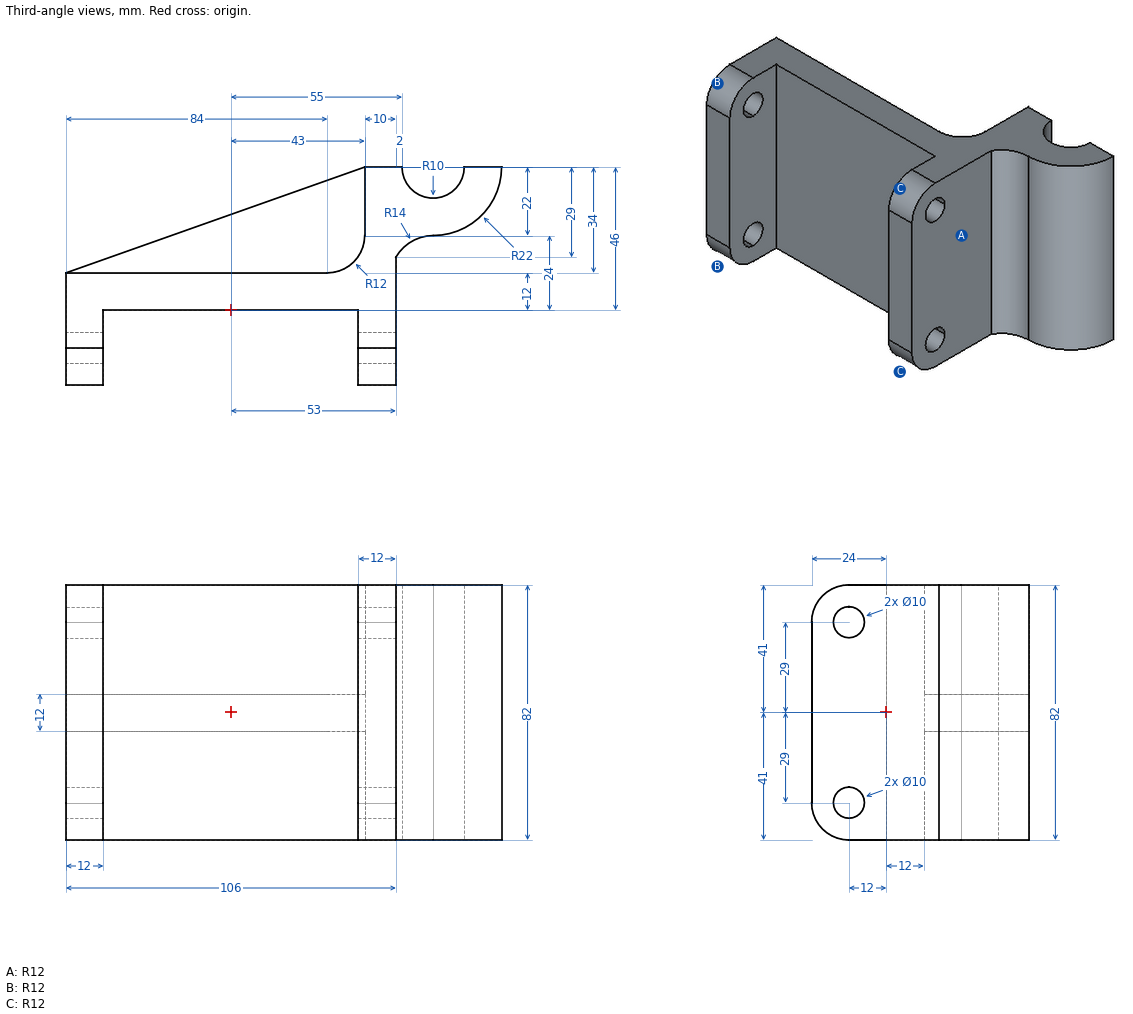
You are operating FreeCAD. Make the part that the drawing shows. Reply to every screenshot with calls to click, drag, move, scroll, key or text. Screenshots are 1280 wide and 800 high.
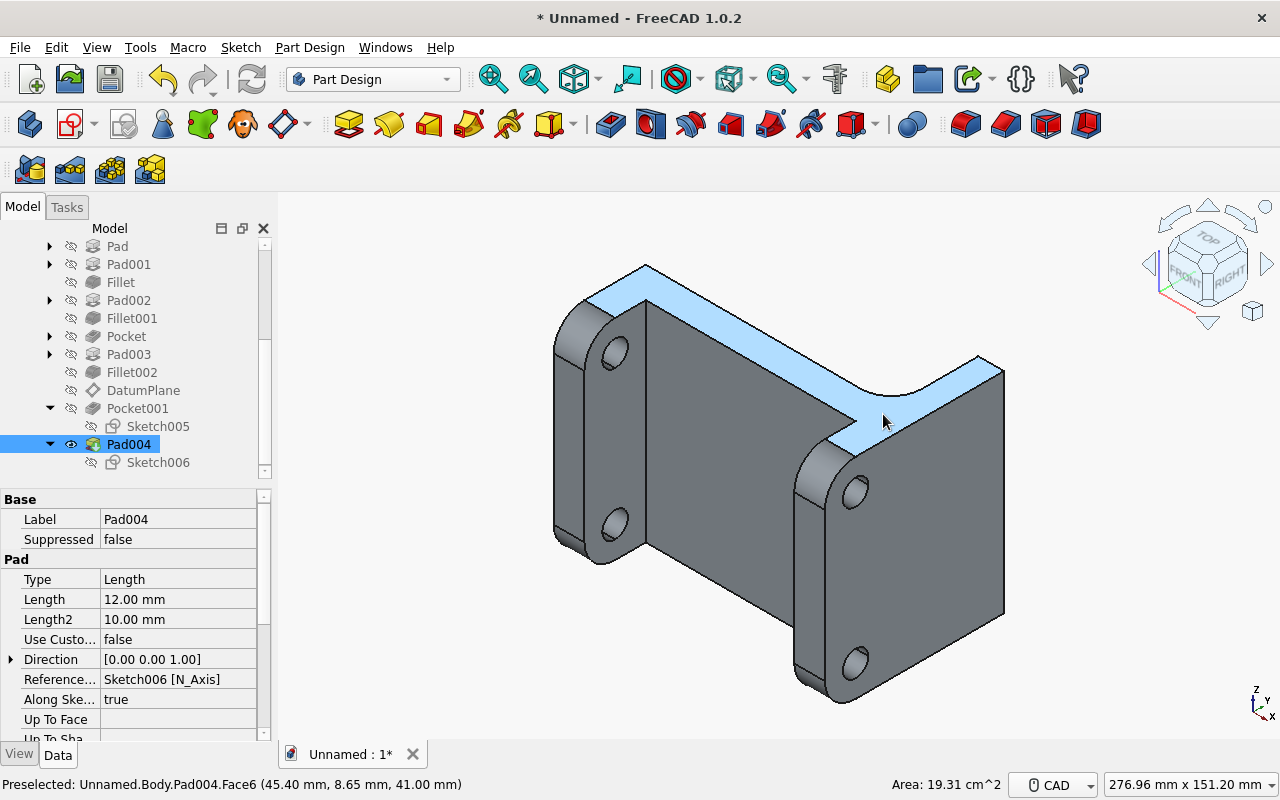
click(70, 124)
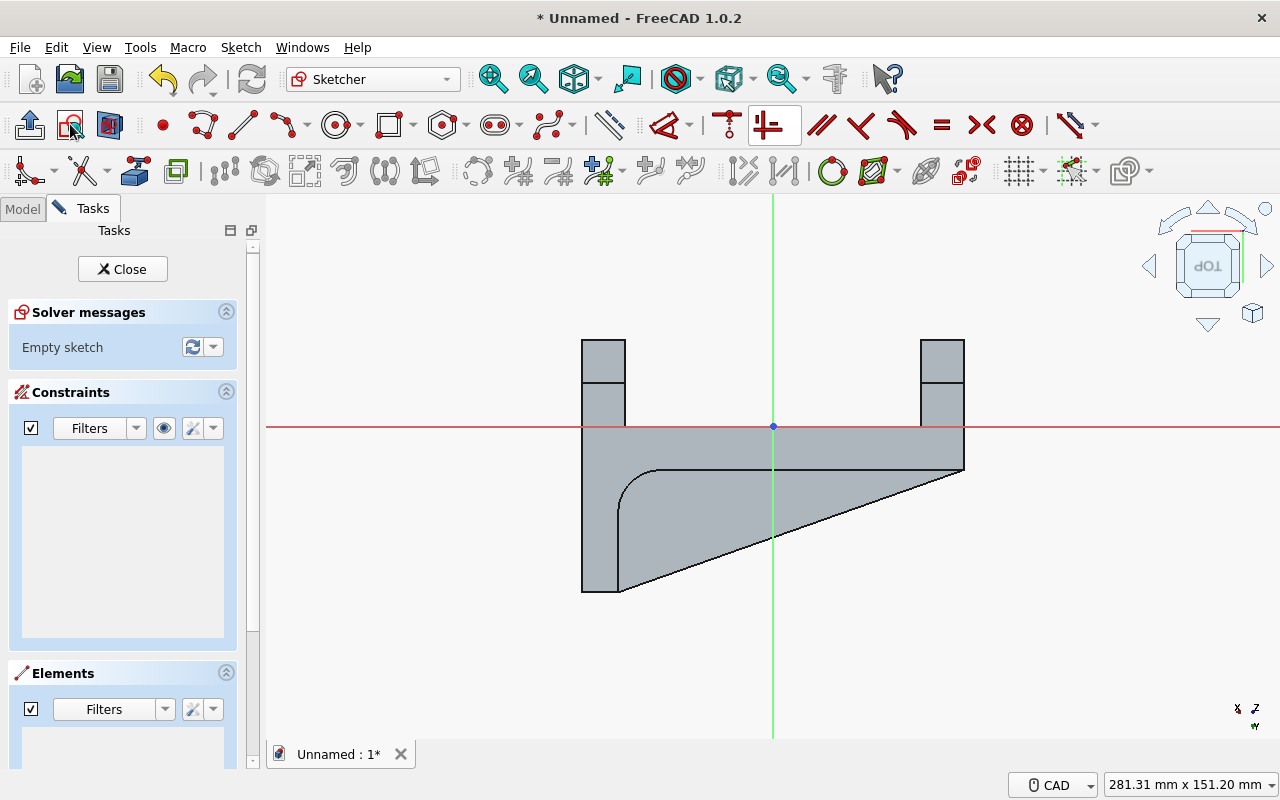
scroll(441, 572, up, 6)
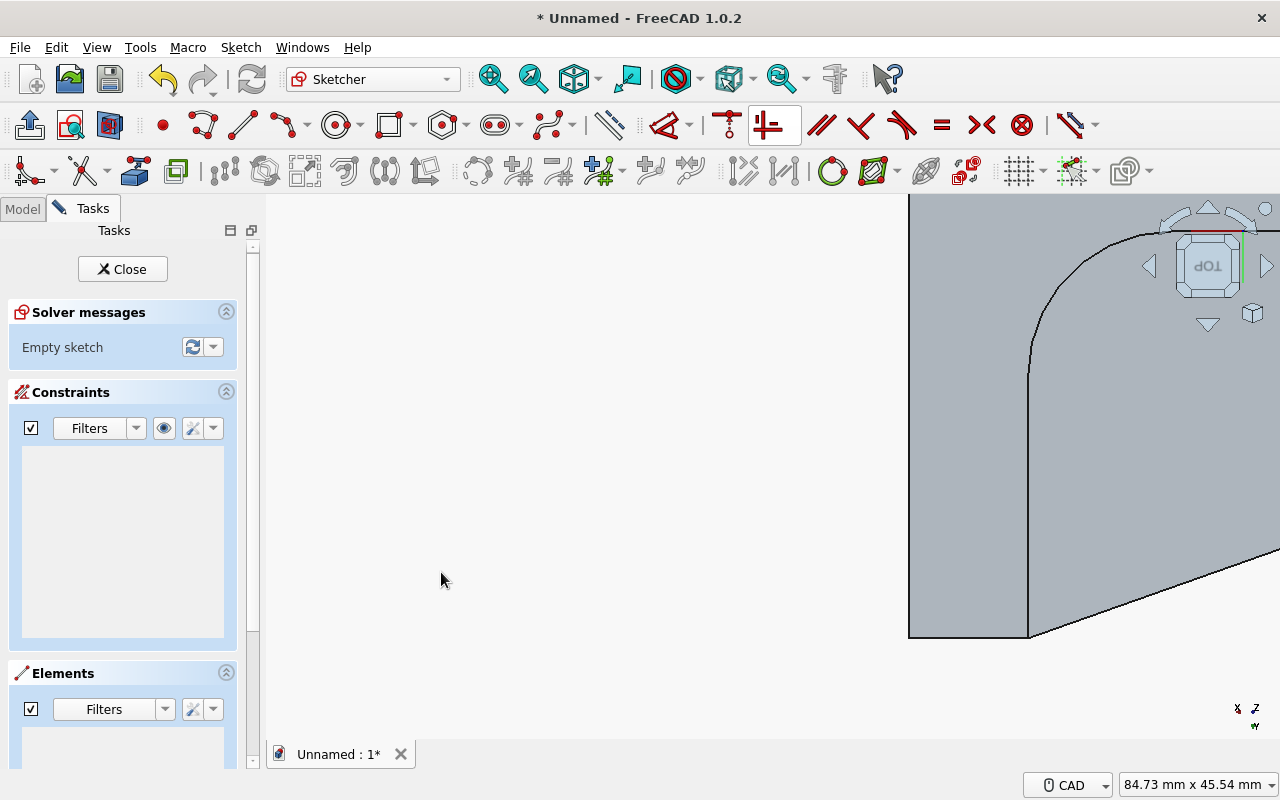
key(g)
key(m)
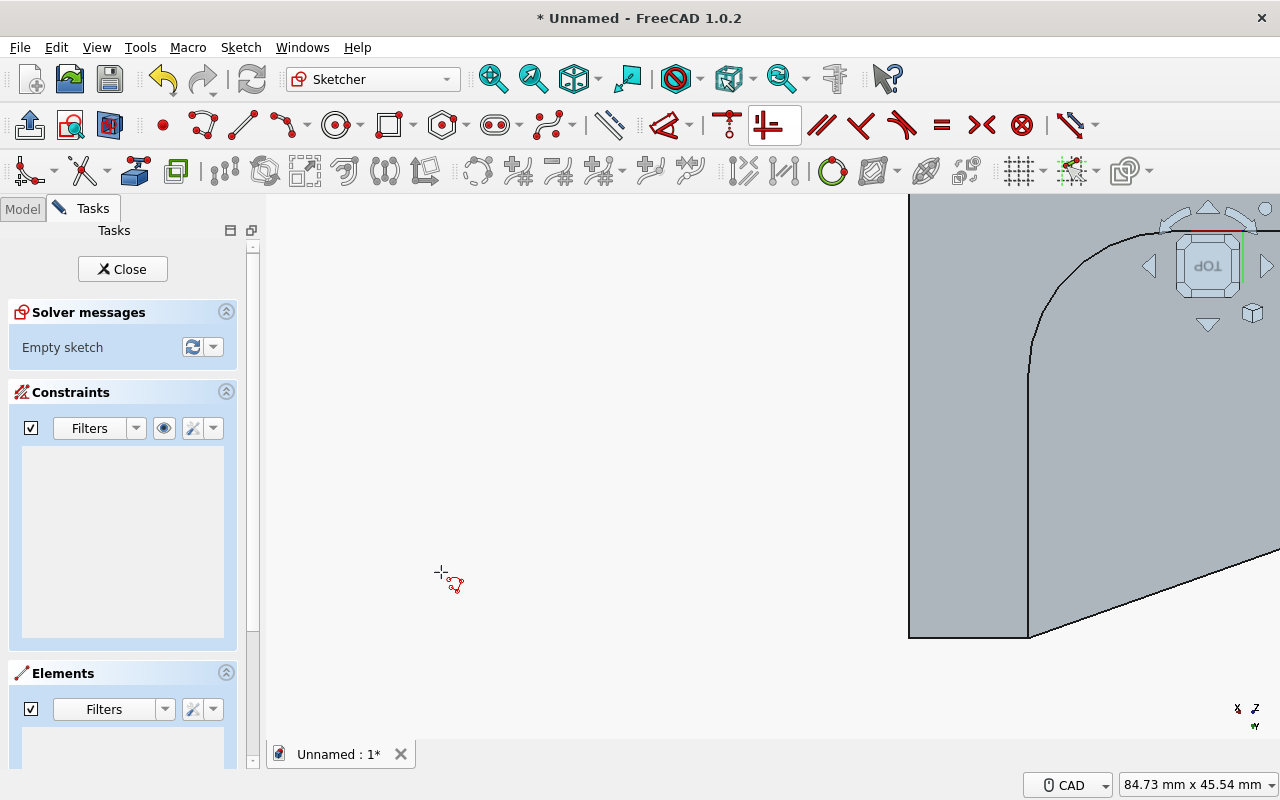
click(885, 638)
click(909, 638)
click(909, 291)
right_click(909, 291)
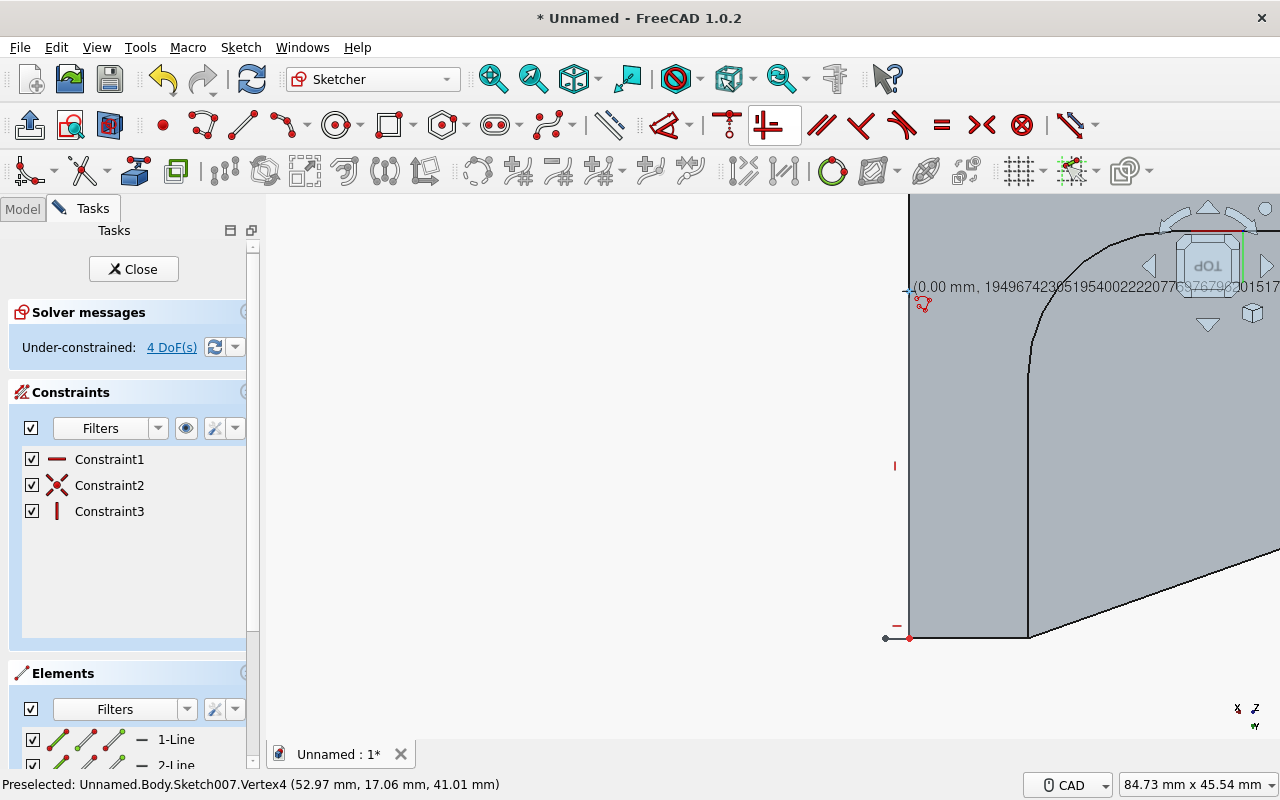
click(244, 126)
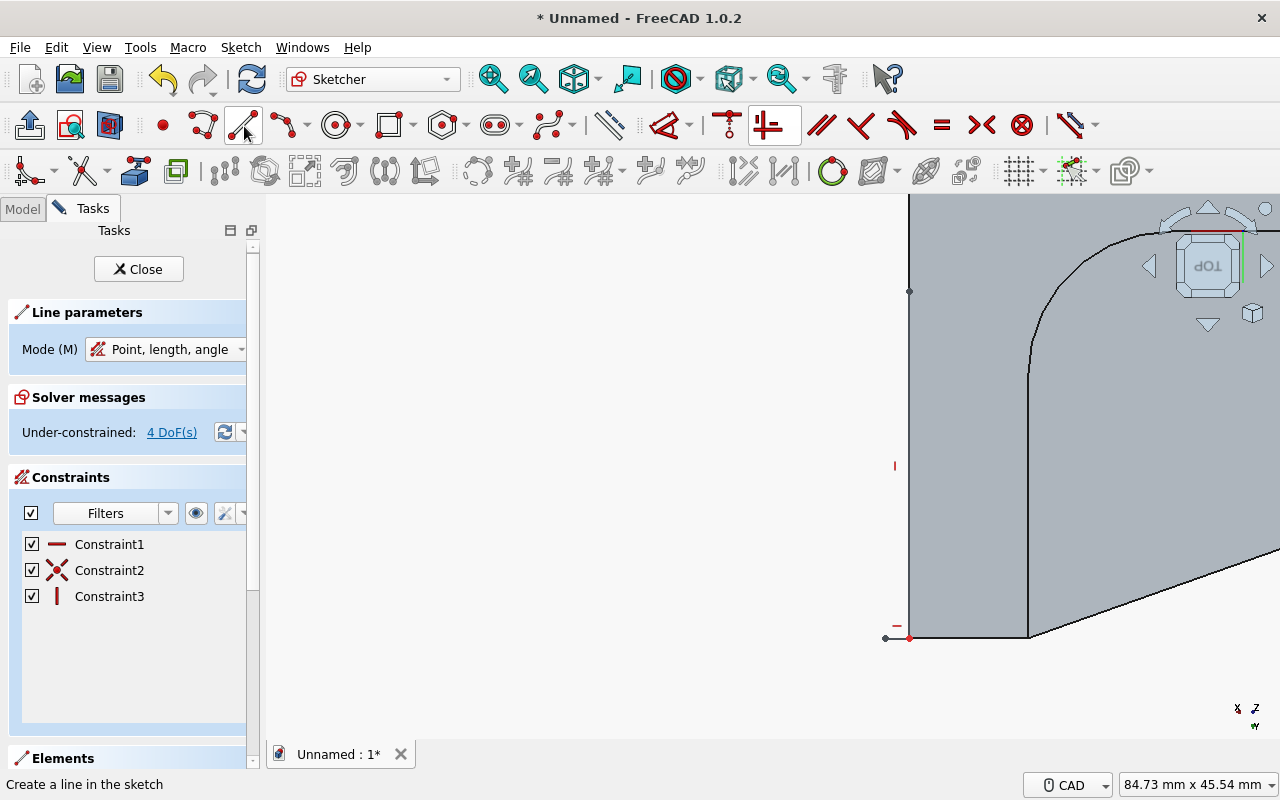
click(502, 638)
click(645, 638)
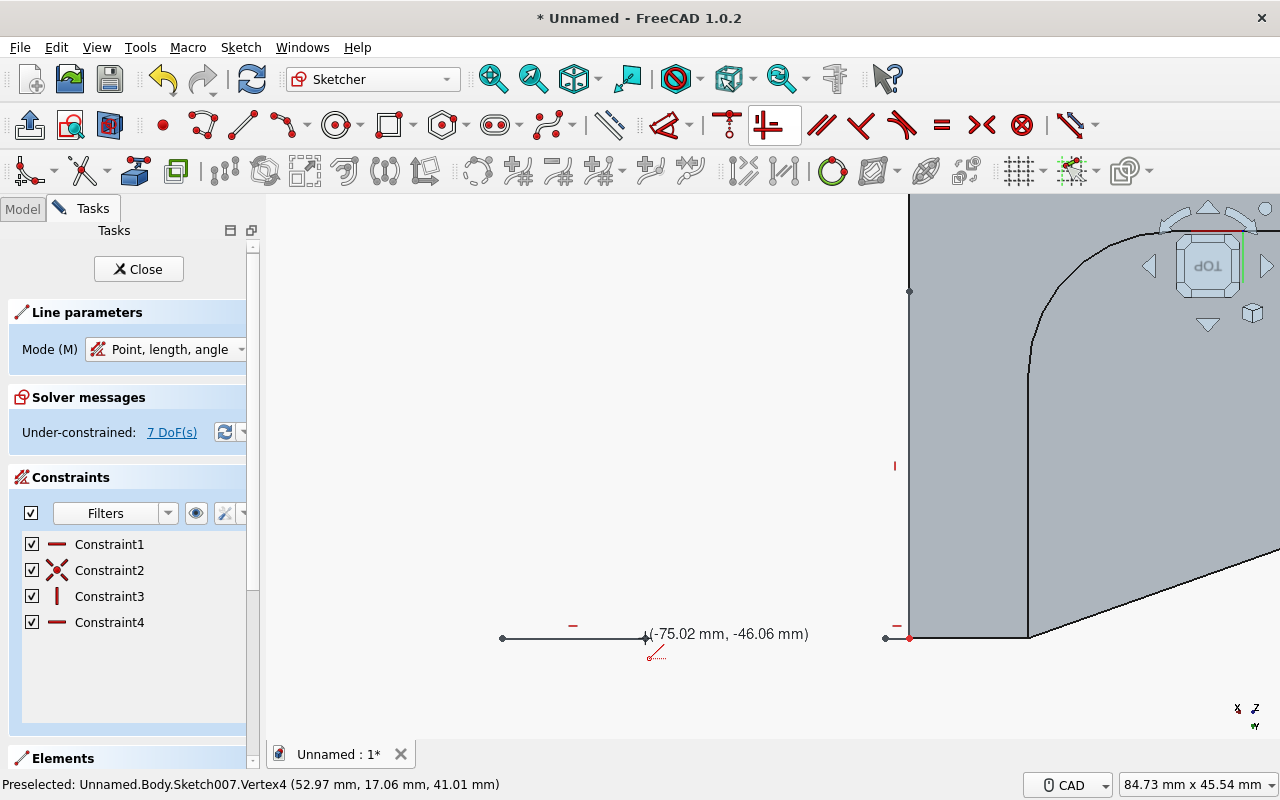
click(284, 126)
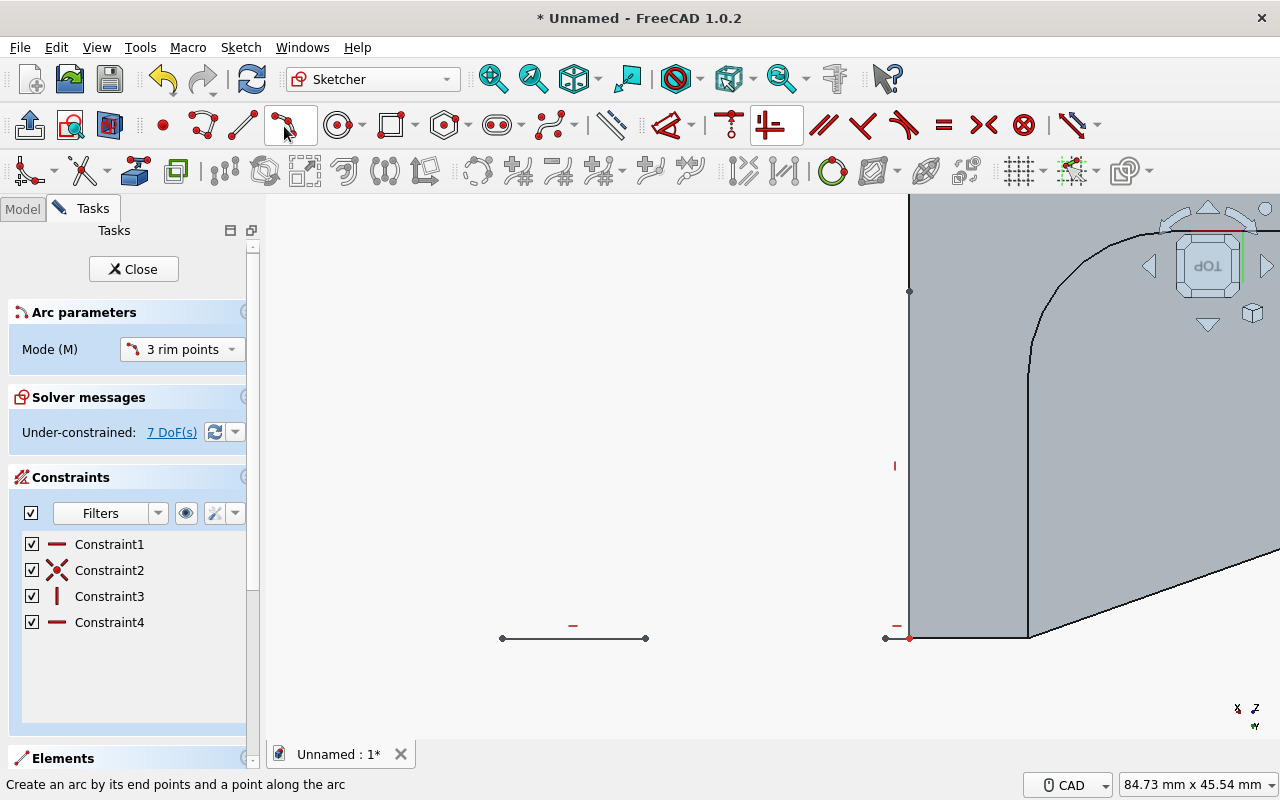
click(909, 292)
click(764, 375)
click(848, 352)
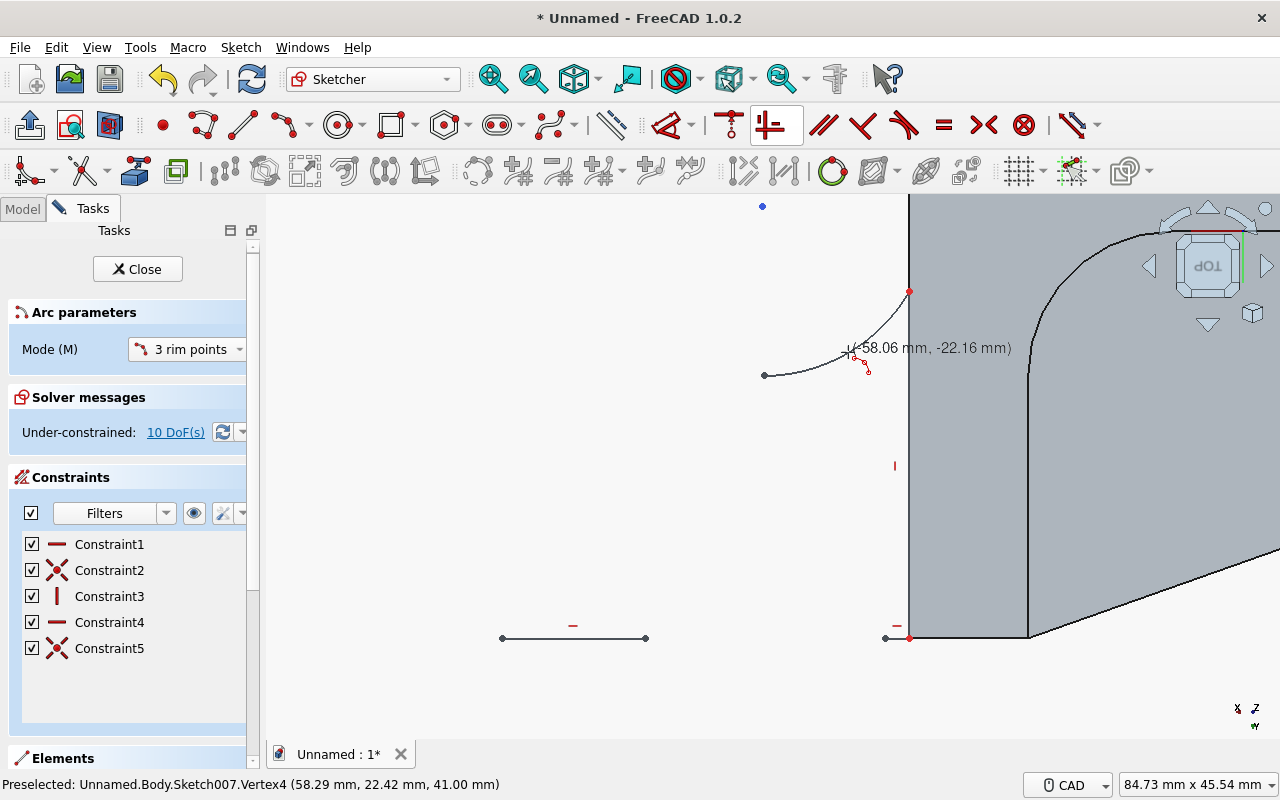
click(764, 376)
click(502, 639)
click(578, 452)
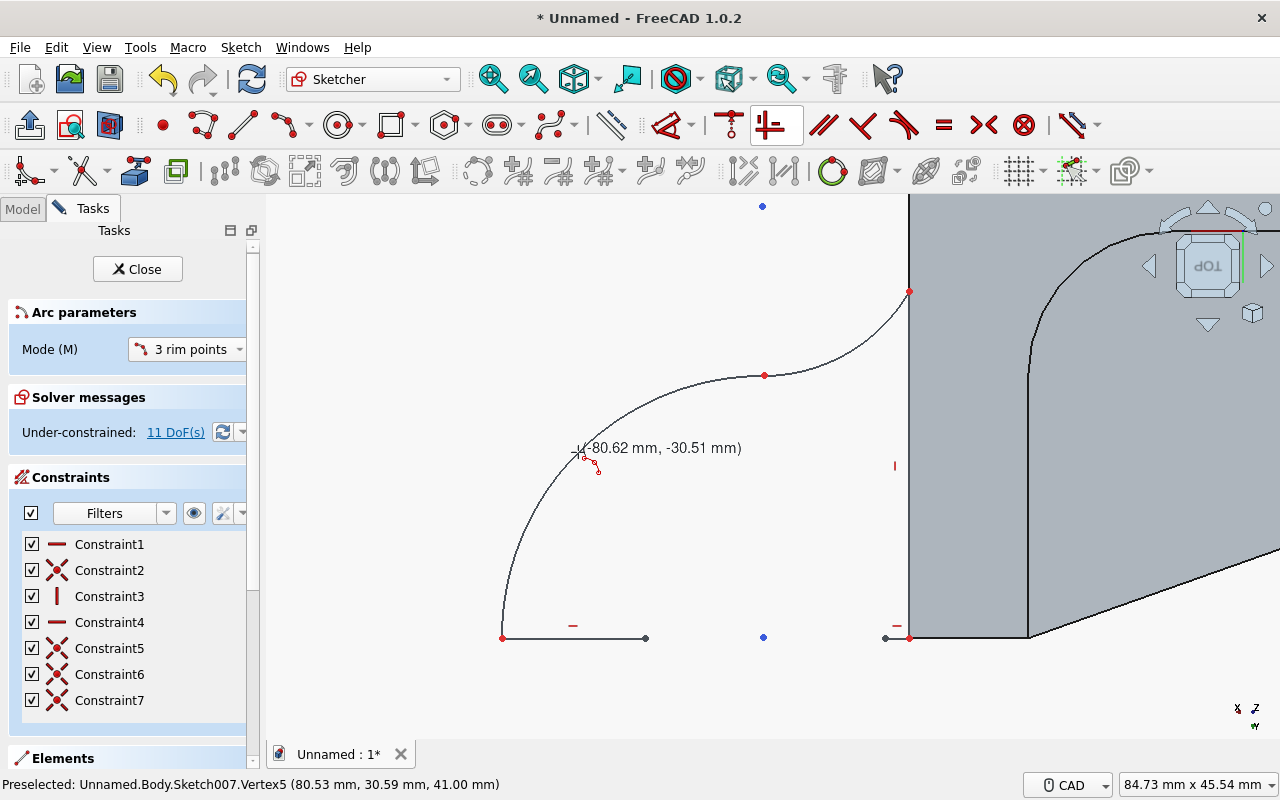
click(645, 639)